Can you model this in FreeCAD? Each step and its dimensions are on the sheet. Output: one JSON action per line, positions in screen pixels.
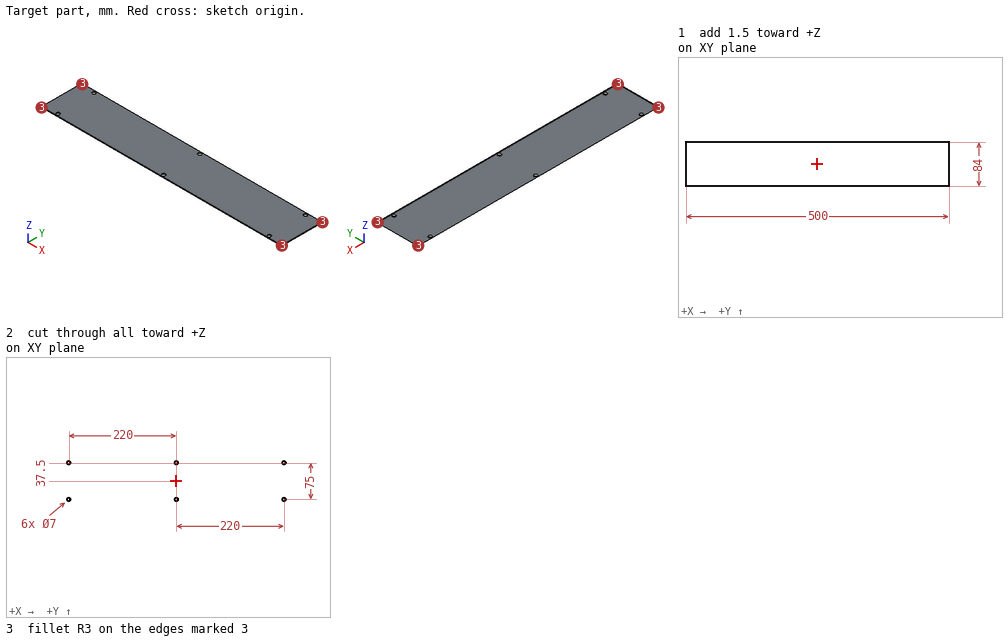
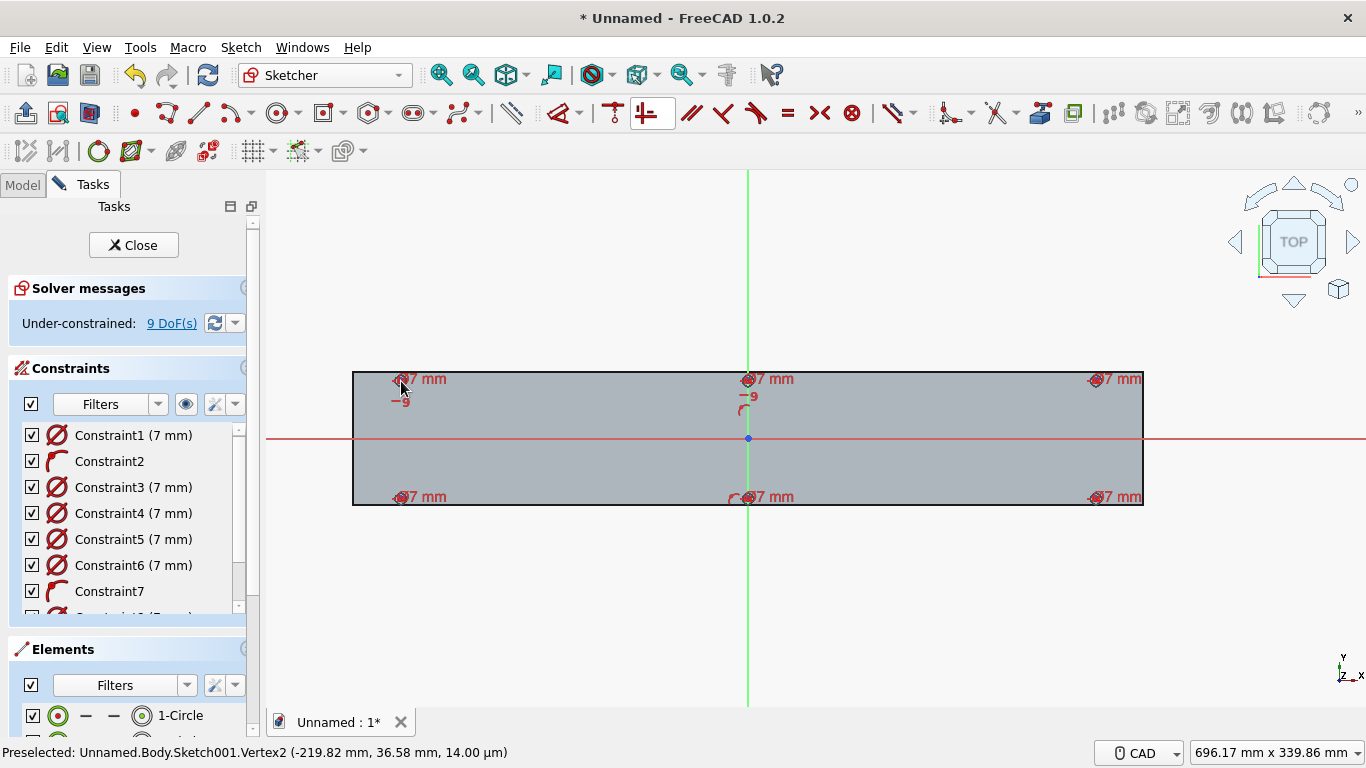
{"action": "left_click", "coordinate": [401, 381]}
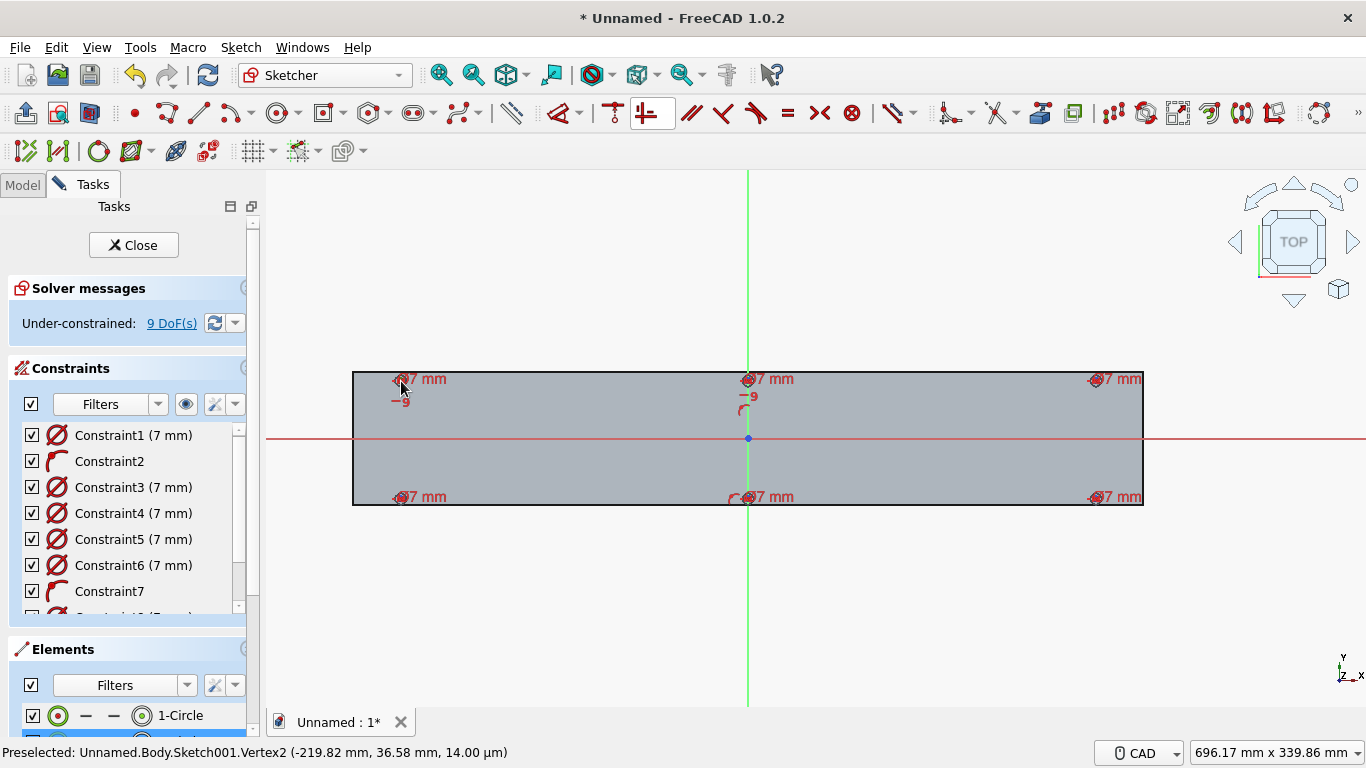
{"action": "left_click", "coordinate": [401, 499]}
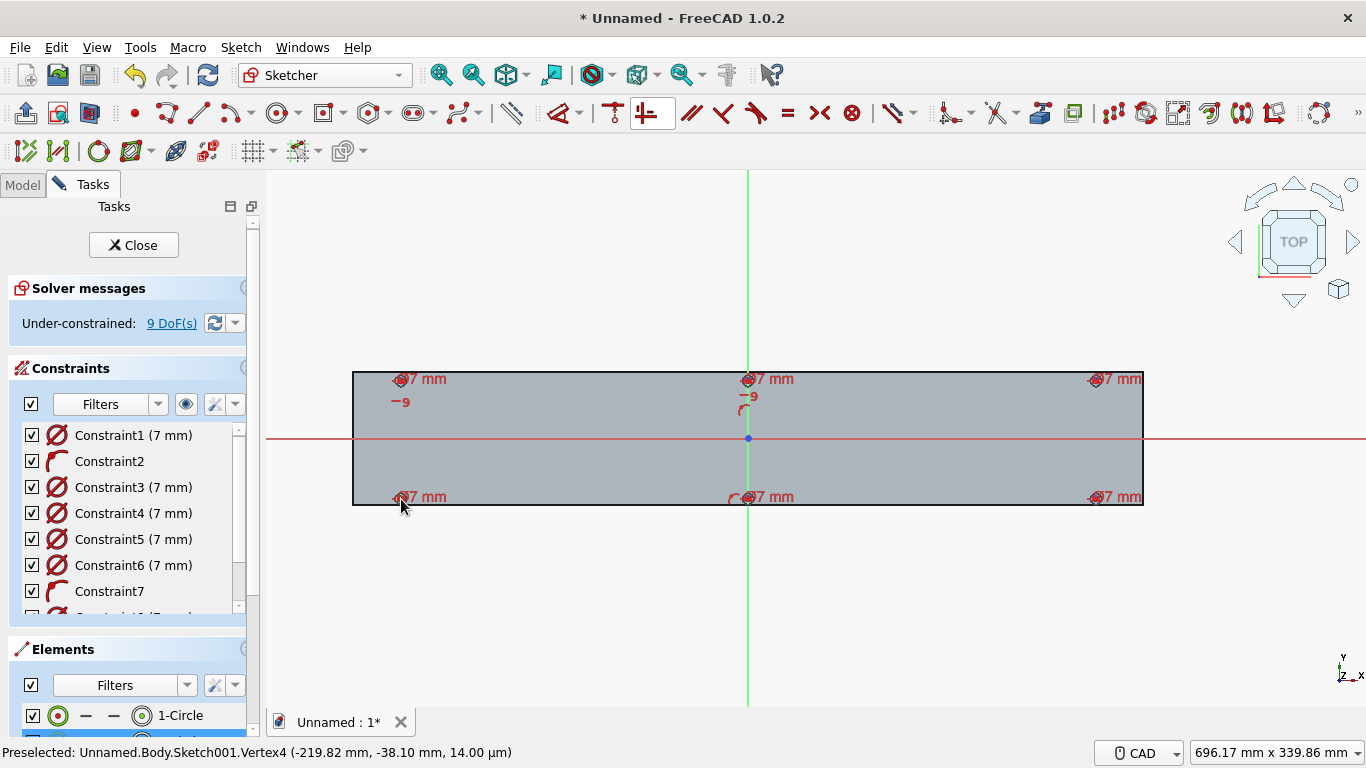
{"action": "left_click", "coordinate": [670, 114]}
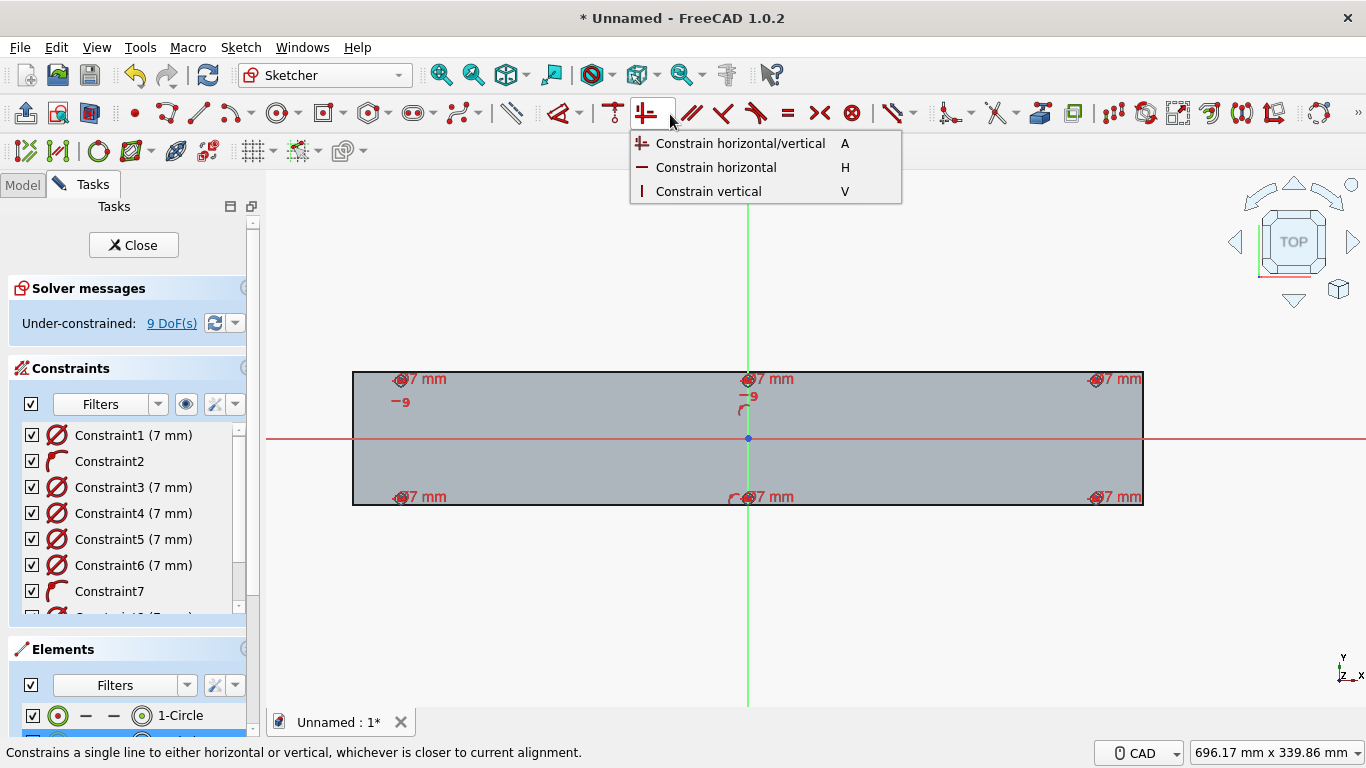
{"action": "left_click", "coordinate": [766, 191]}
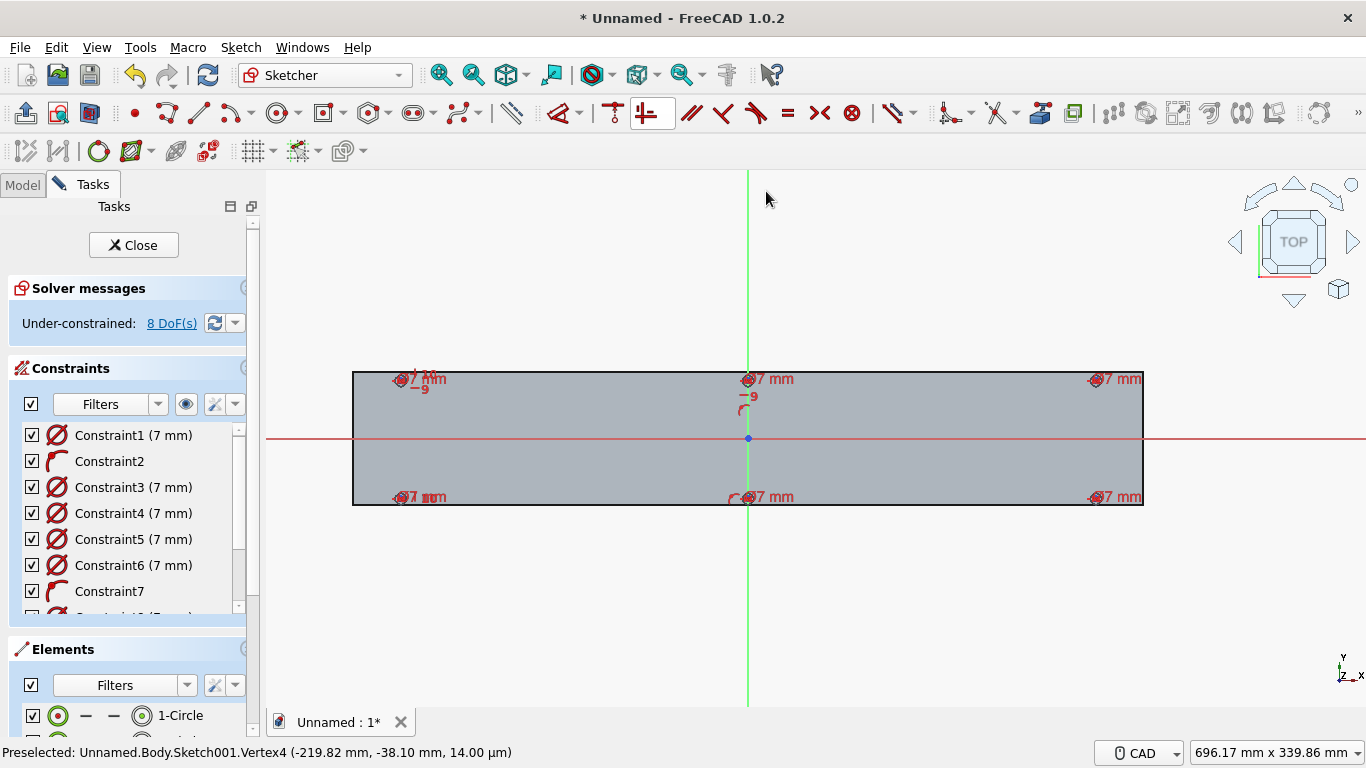
{"action": "left_click", "coordinate": [1096, 499]}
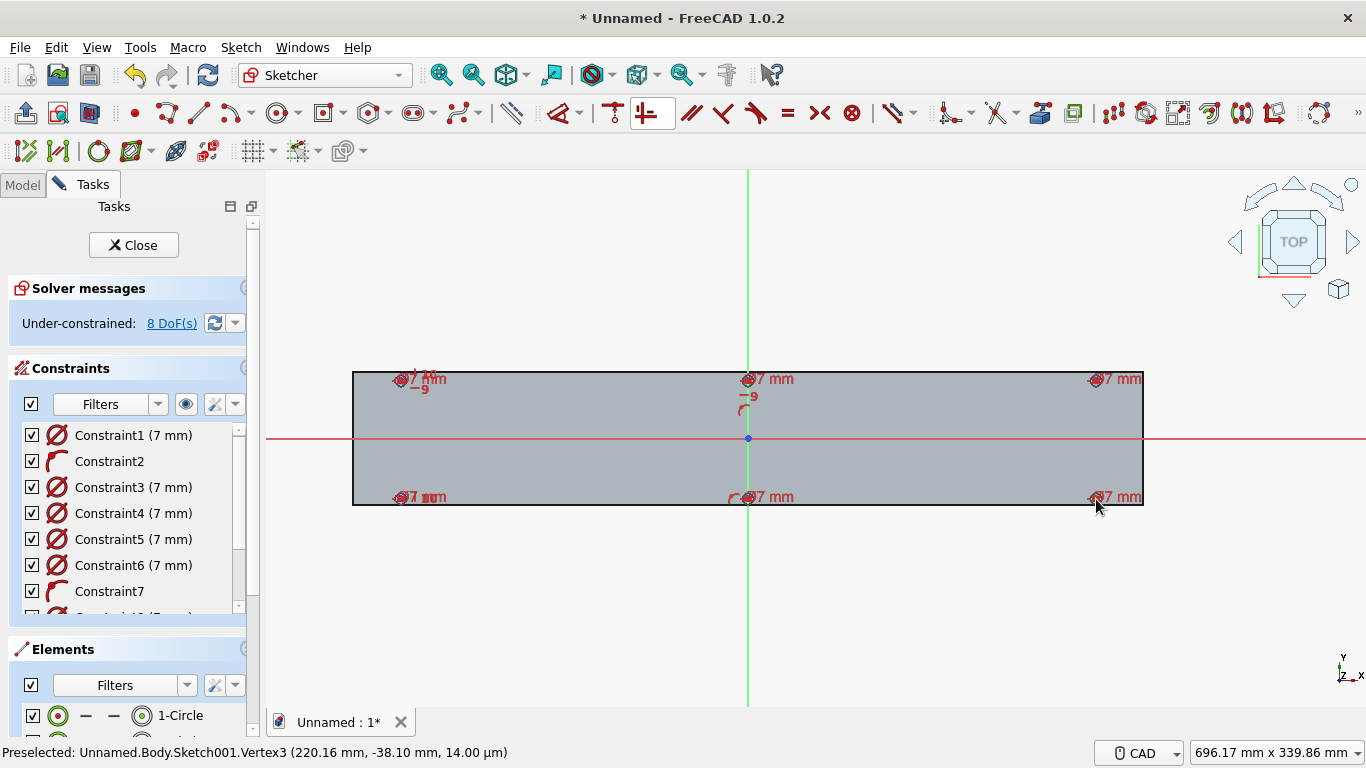
{"action": "left_click", "coordinate": [401, 499]}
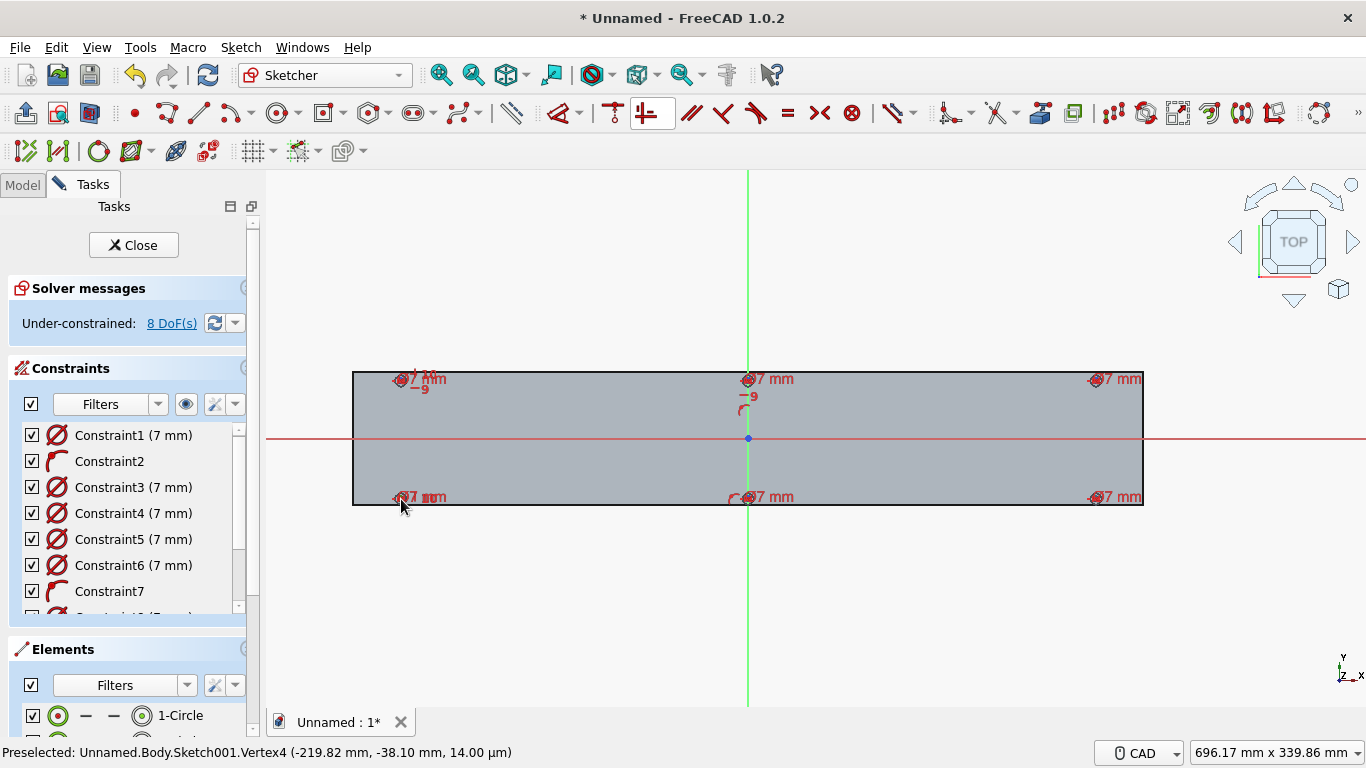
{"action": "left_click", "coordinate": [670, 114]}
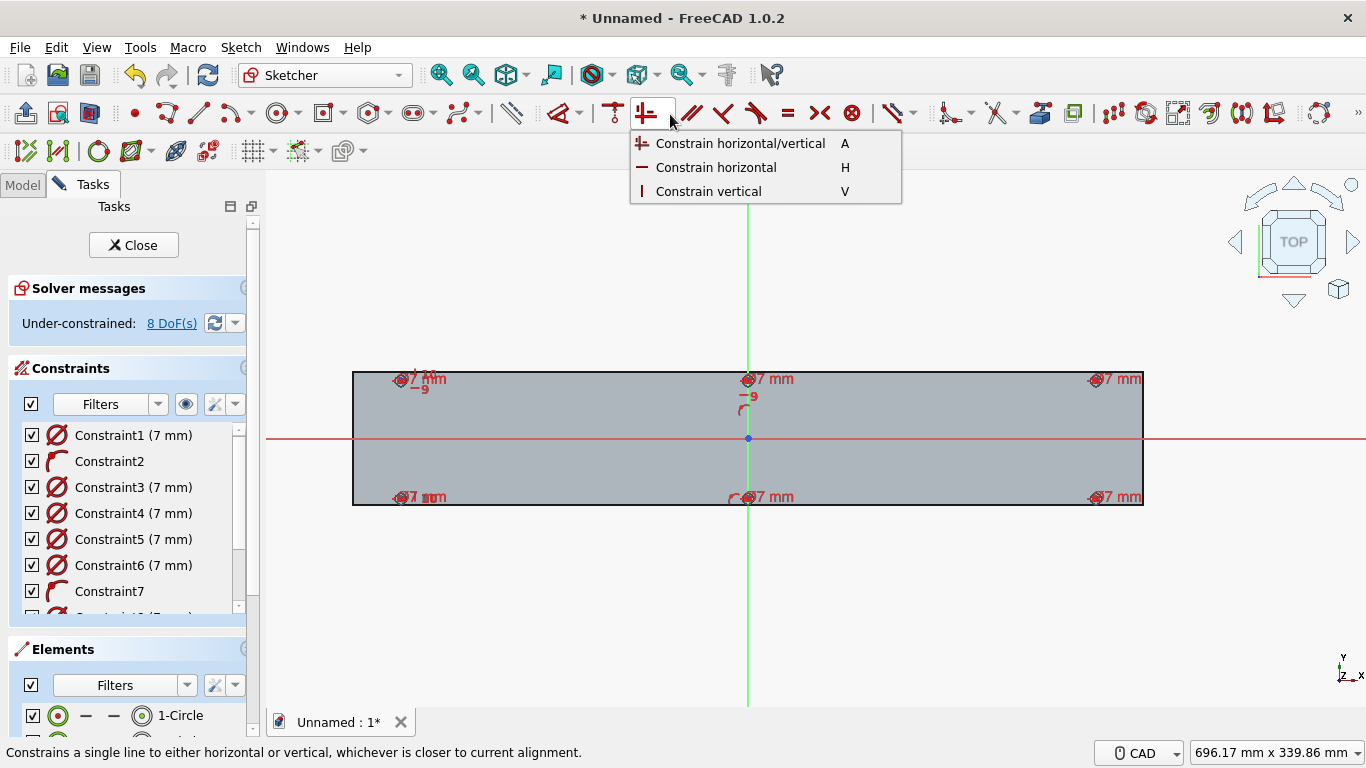
{"action": "left_click", "coordinate": [766, 167]}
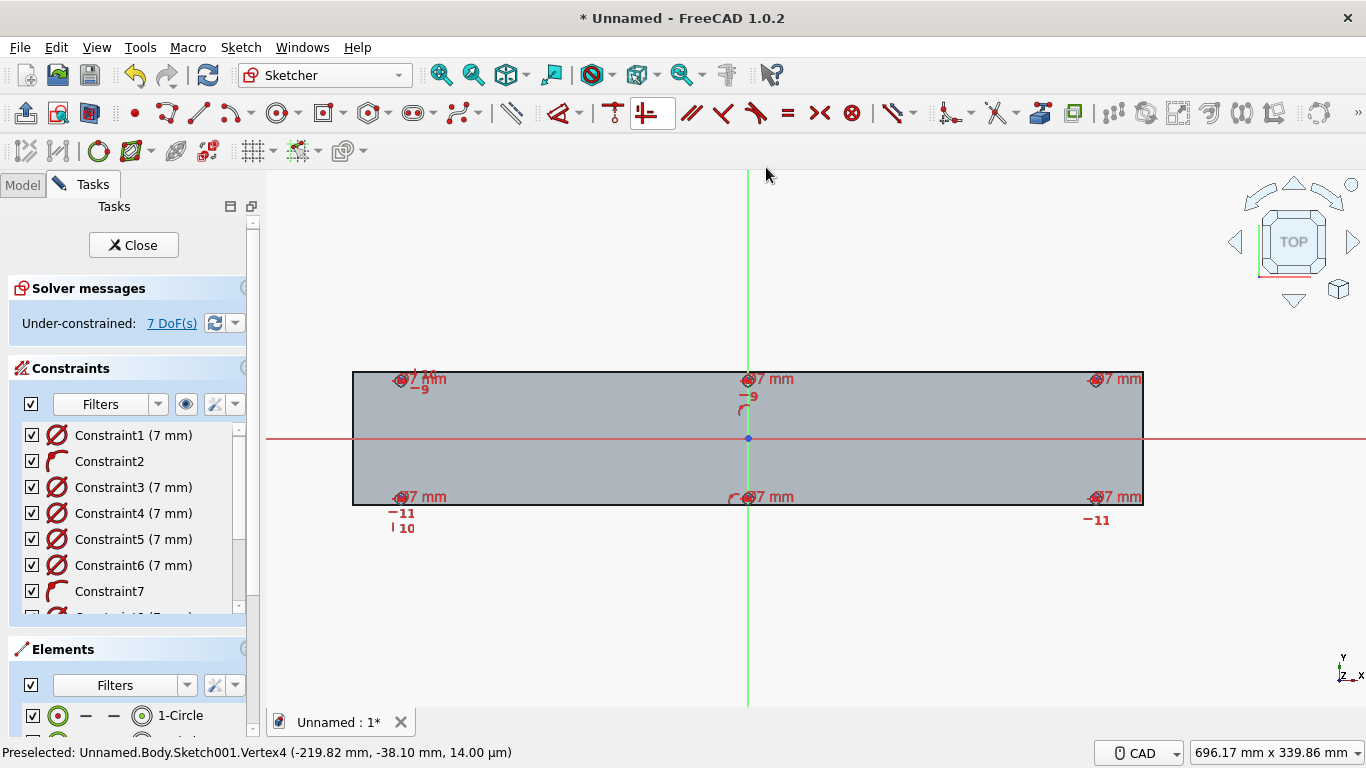
{"action": "left_click", "coordinate": [1096, 499]}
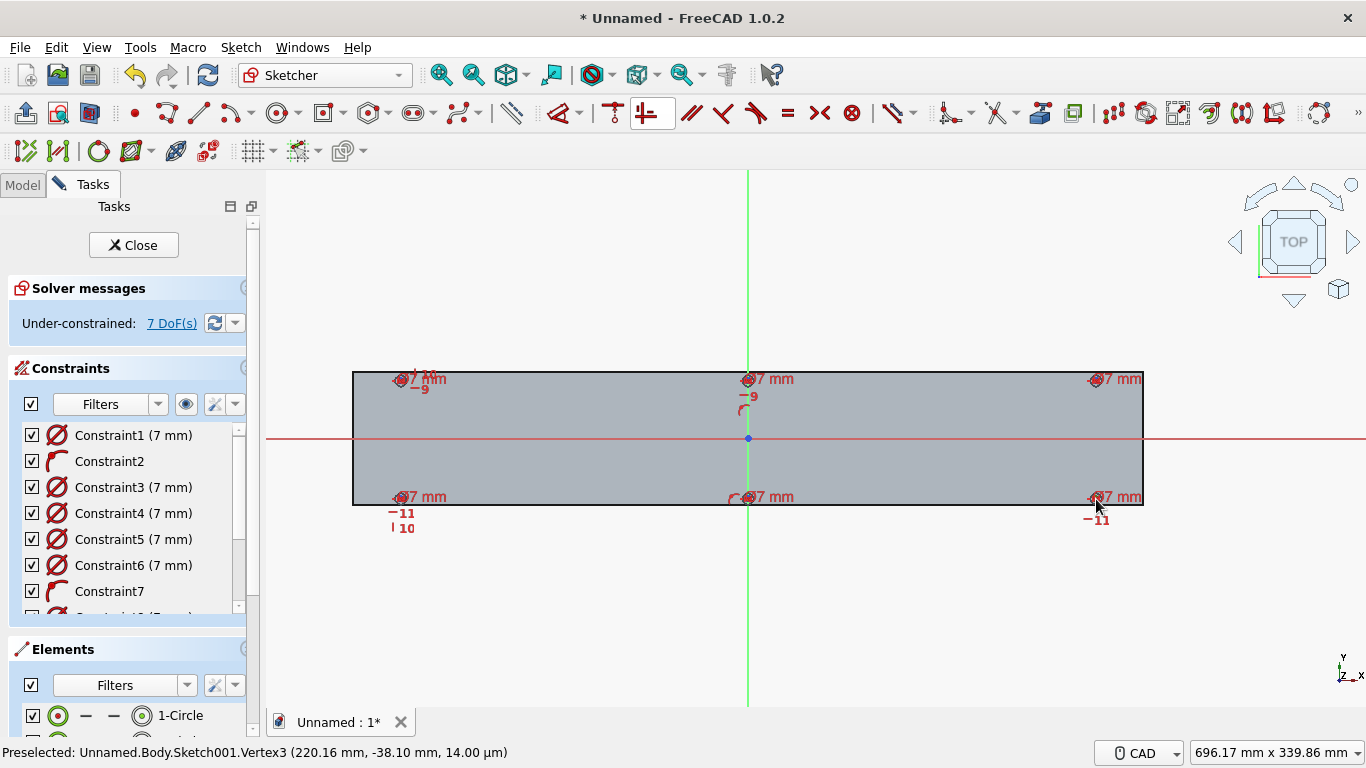
{"action": "left_click", "coordinate": [748, 499]}